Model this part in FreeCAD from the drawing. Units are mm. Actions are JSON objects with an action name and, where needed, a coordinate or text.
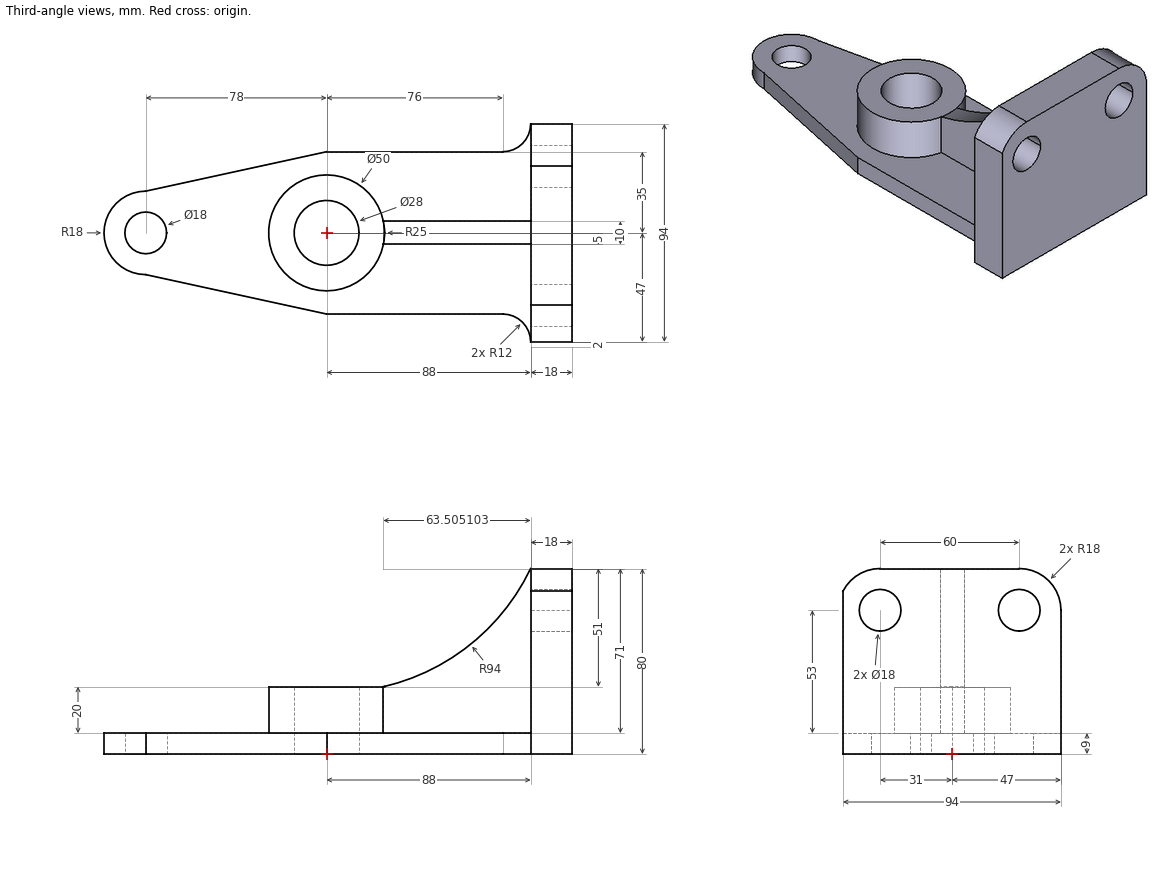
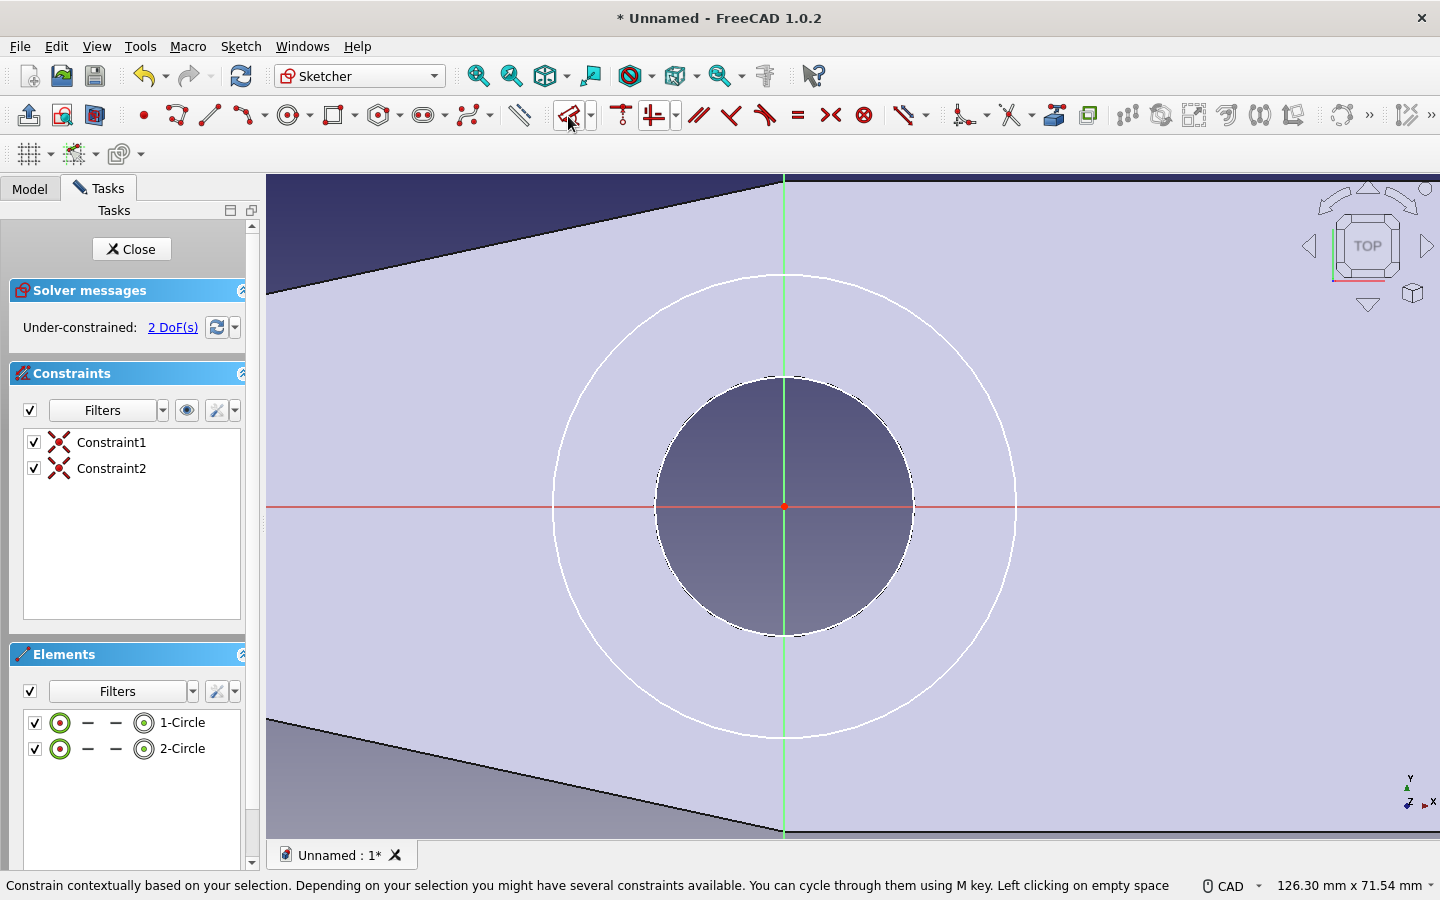
{"action": "left_click", "coordinate": [948, 342]}
{"action": "left_click", "coordinate": [971, 319]}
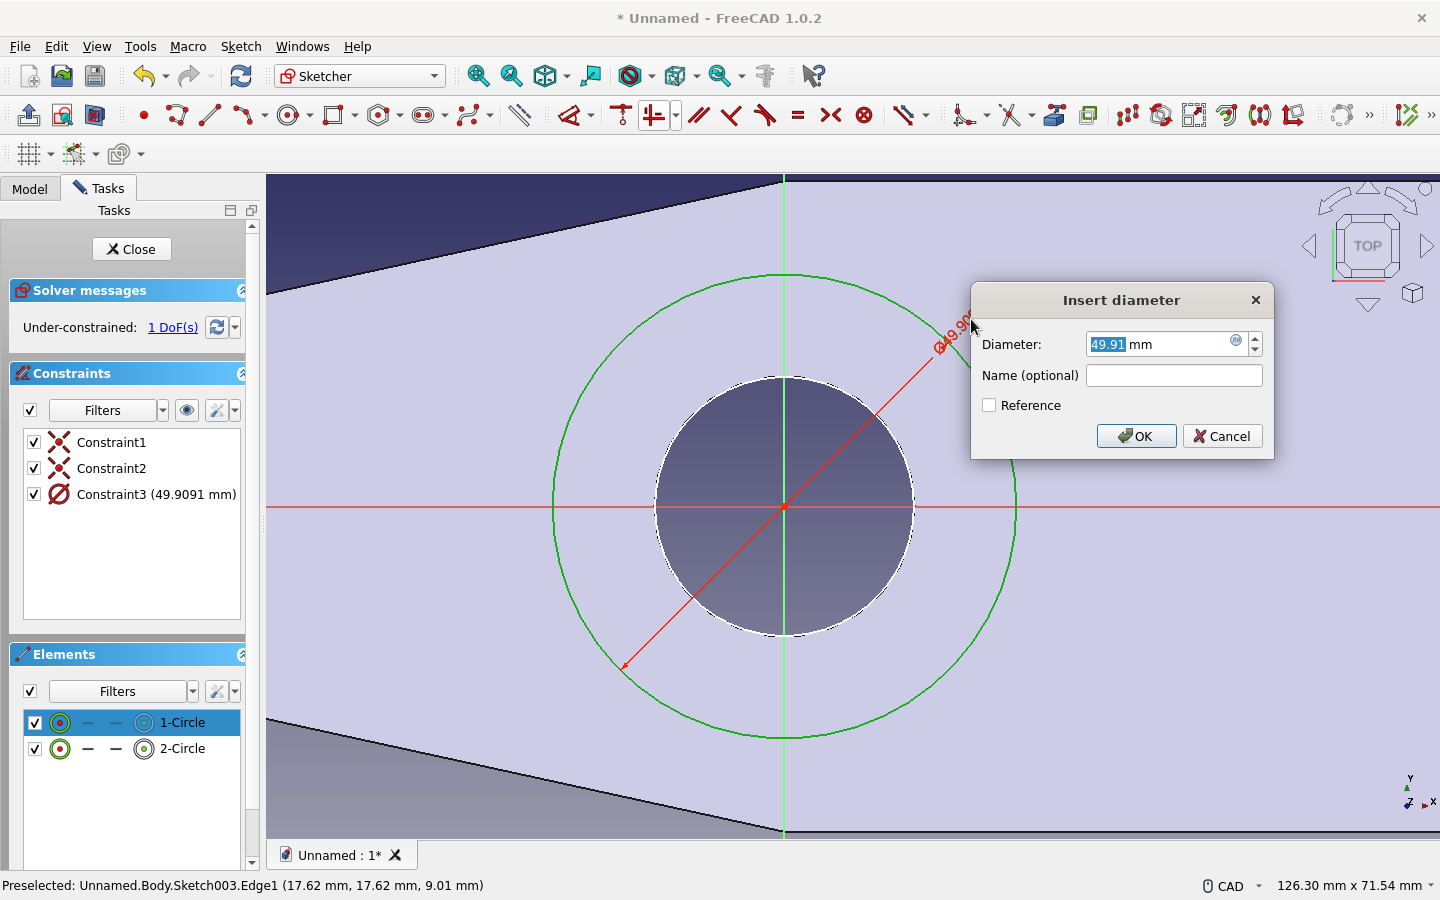
{"action": "type", "text": "50"}
{"action": "key", "text": "Return"}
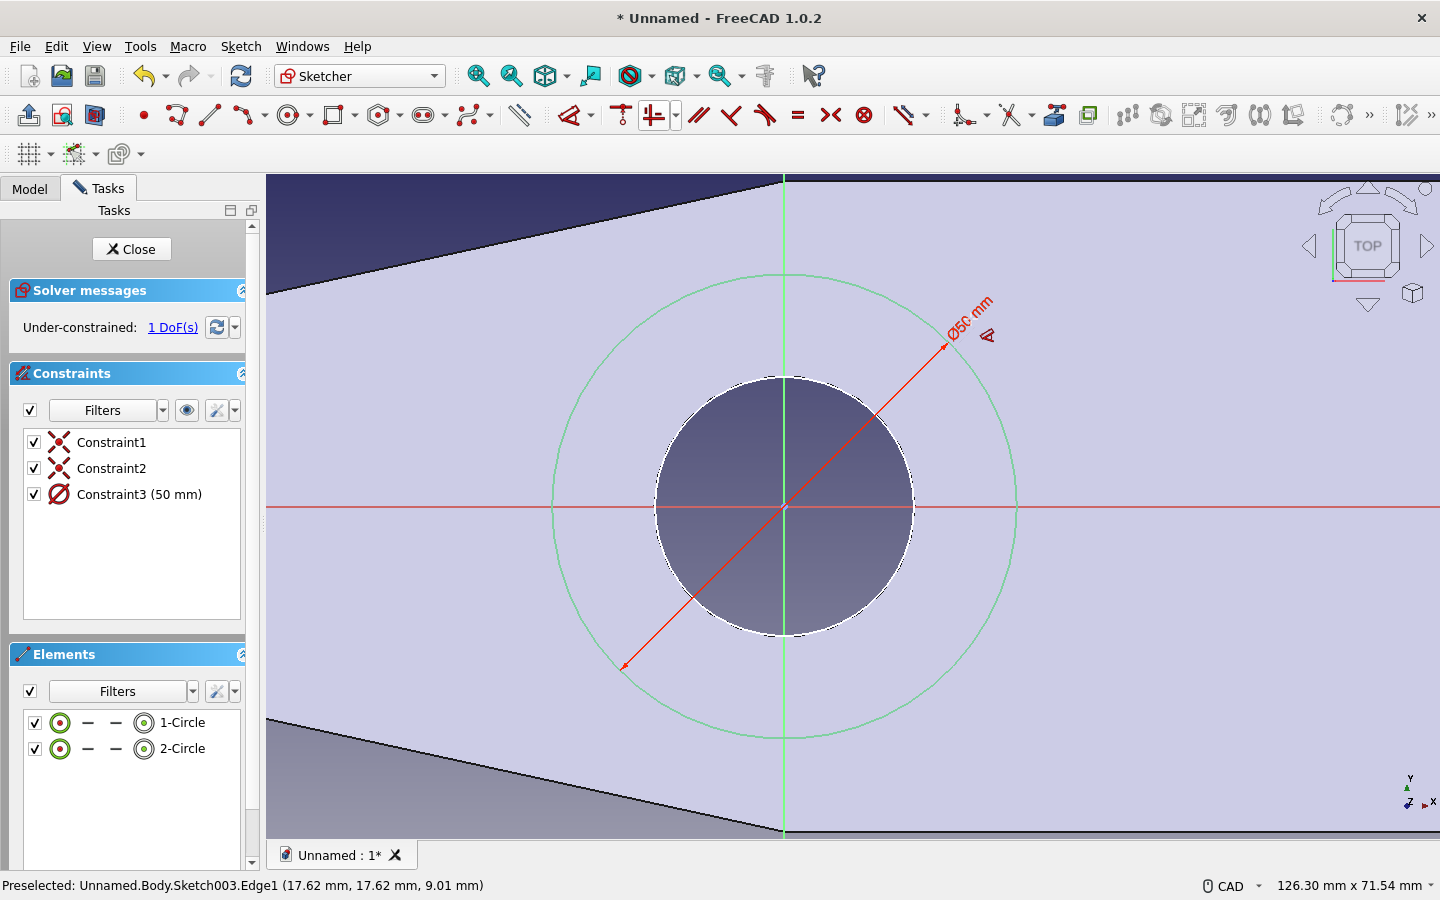
{"action": "left_click", "coordinate": [876, 415]}
{"action": "left_click", "coordinate": [899, 392]}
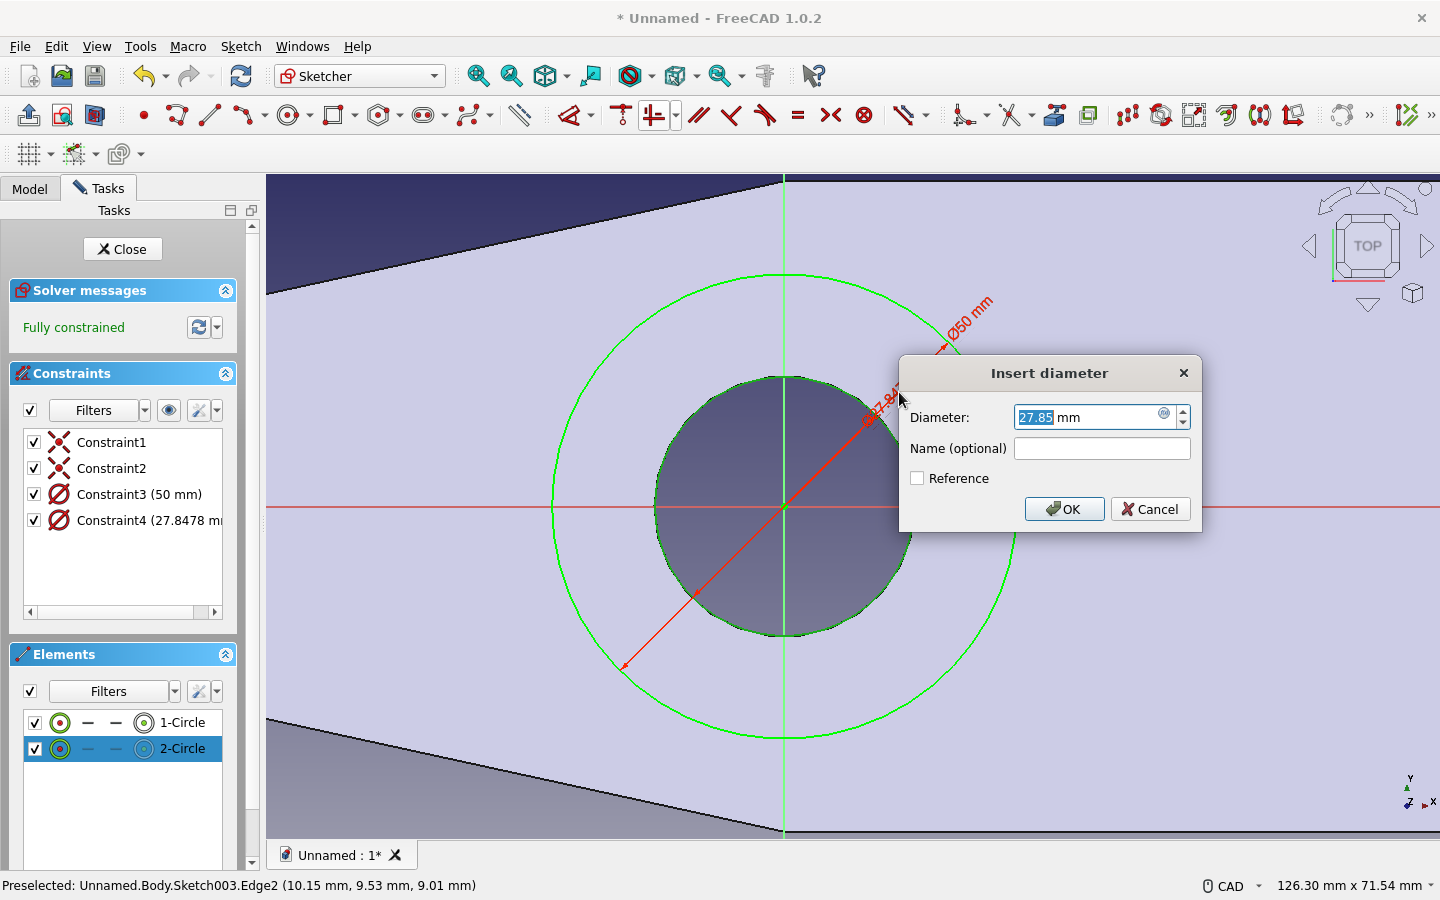
{"action": "type", "text": "28"}
{"action": "key", "text": "Return"}
{"action": "key", "text": "Escape"}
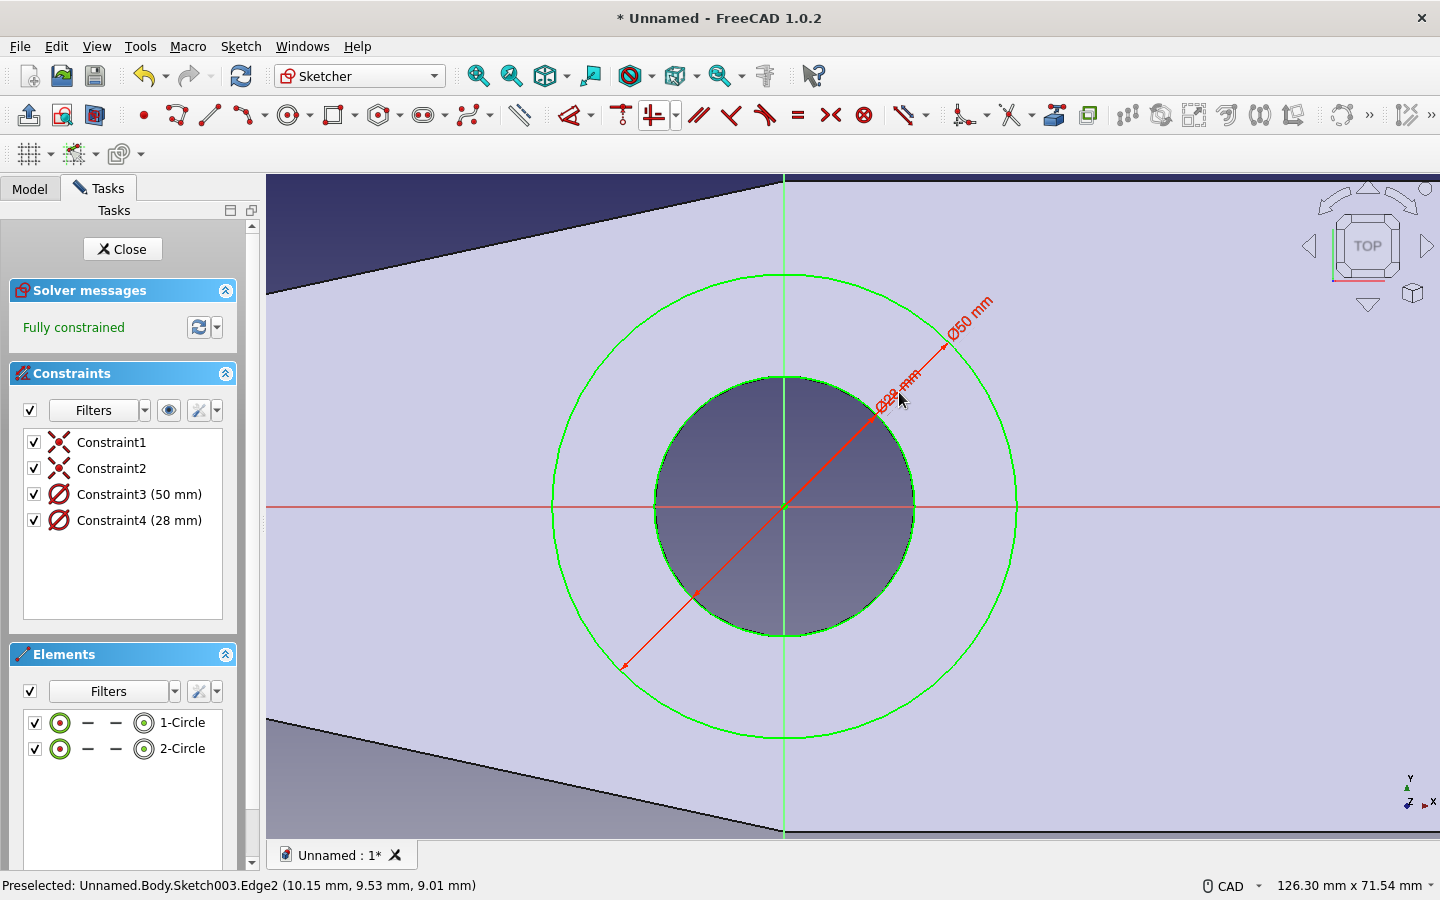
{"action": "left_click", "coordinate": [123, 249]}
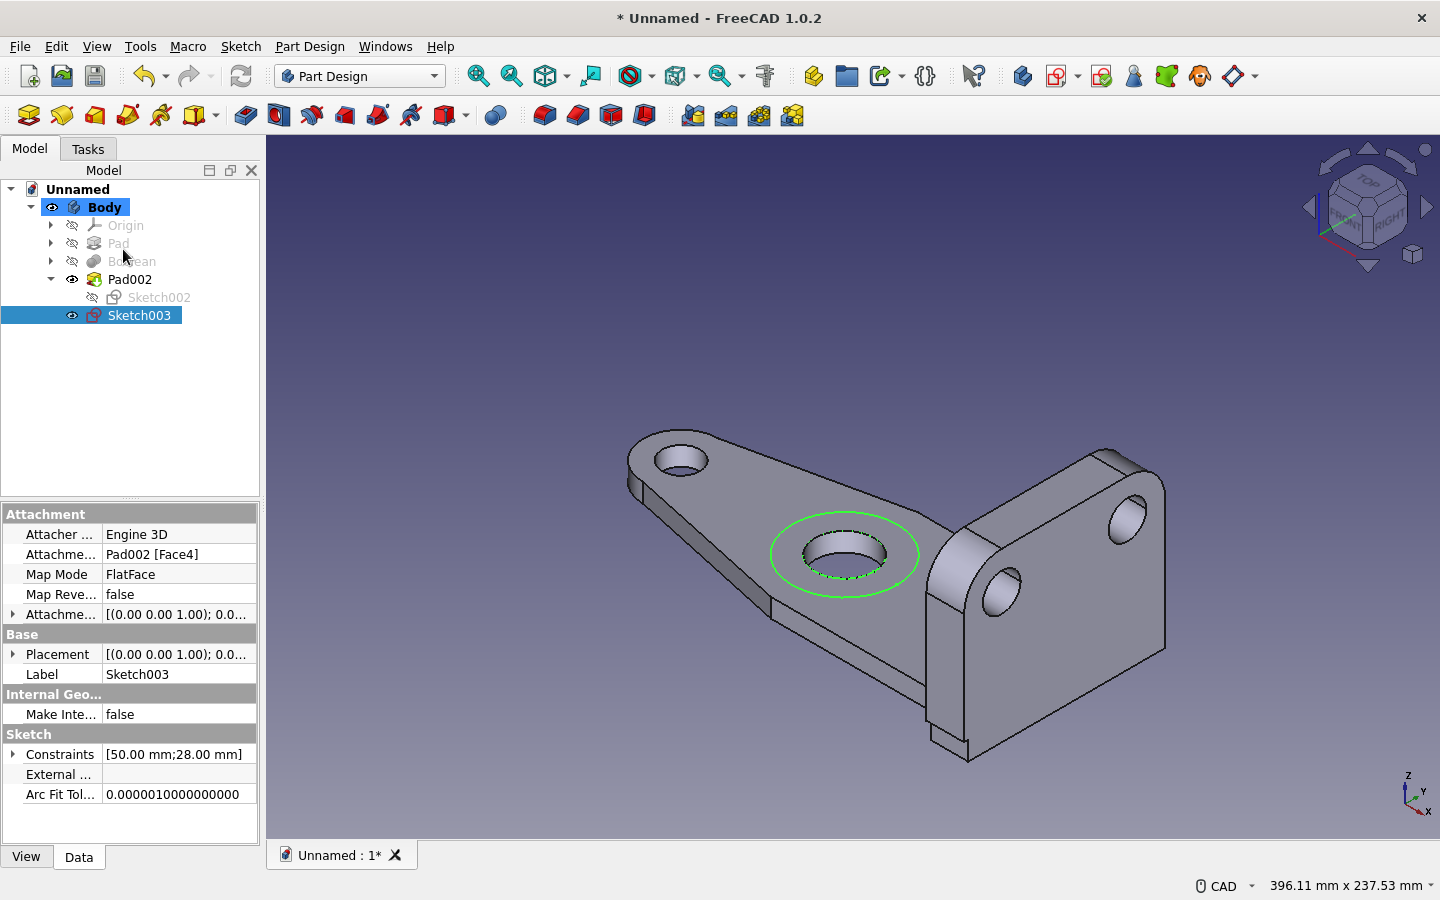
{"action": "left_click", "coordinate": [29, 116]}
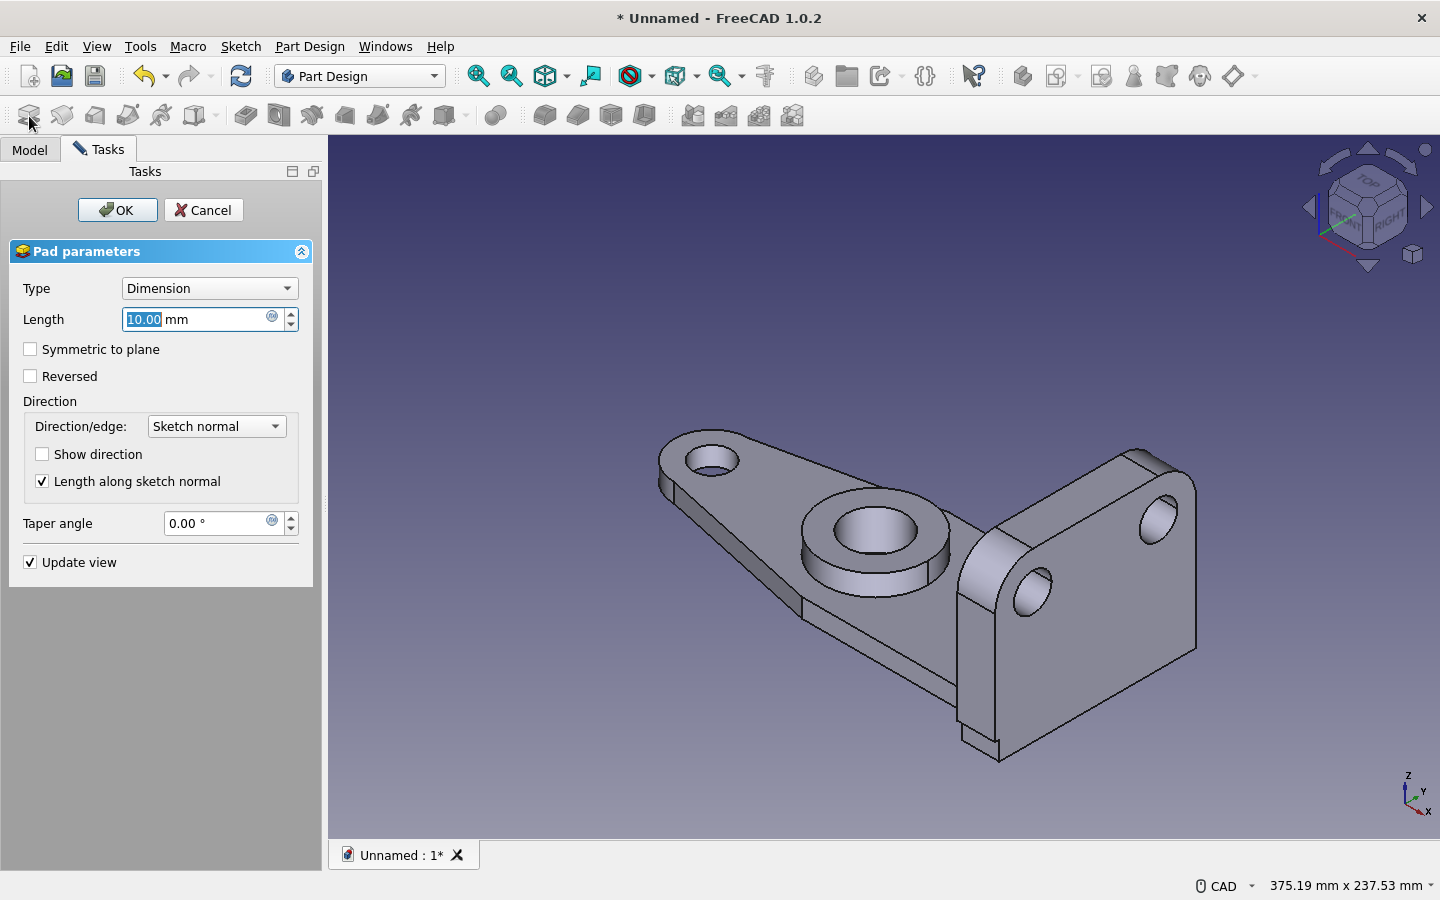
{"action": "type", "text": "20"}
{"action": "key", "text": "Tab"}